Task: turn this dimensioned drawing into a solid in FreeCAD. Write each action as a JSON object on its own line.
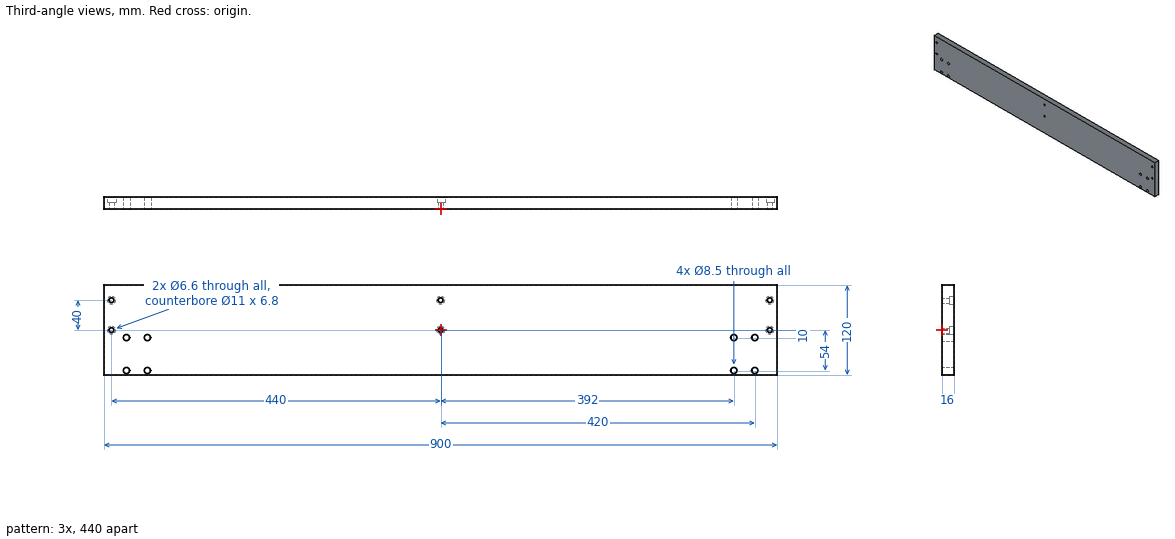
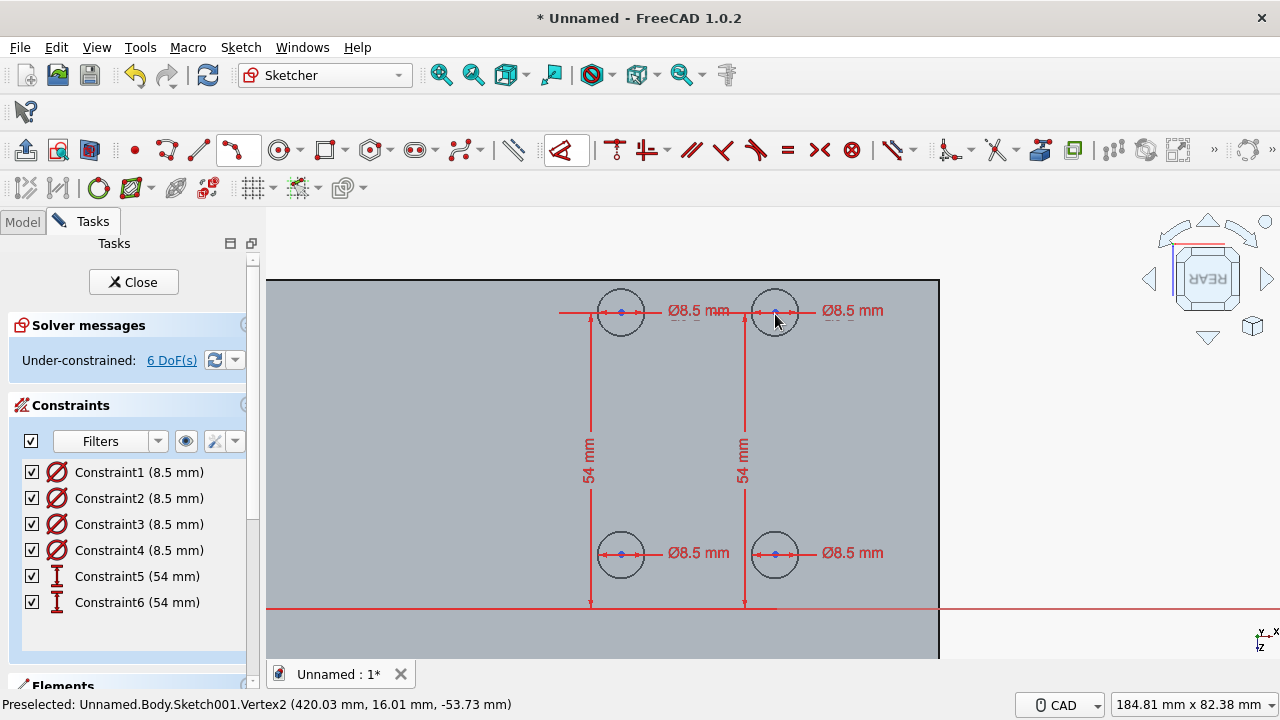
{"action": "left_click", "coordinate": [621, 555]}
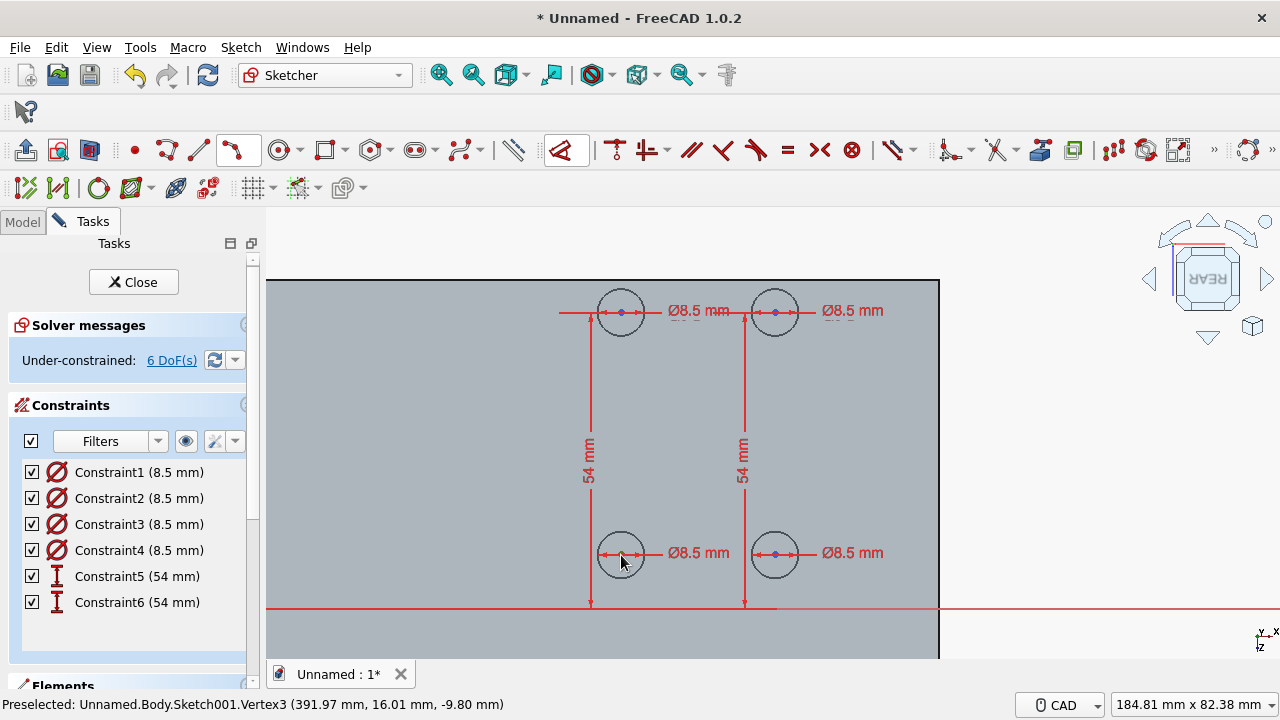
{"action": "left_click", "coordinate": [584, 150]}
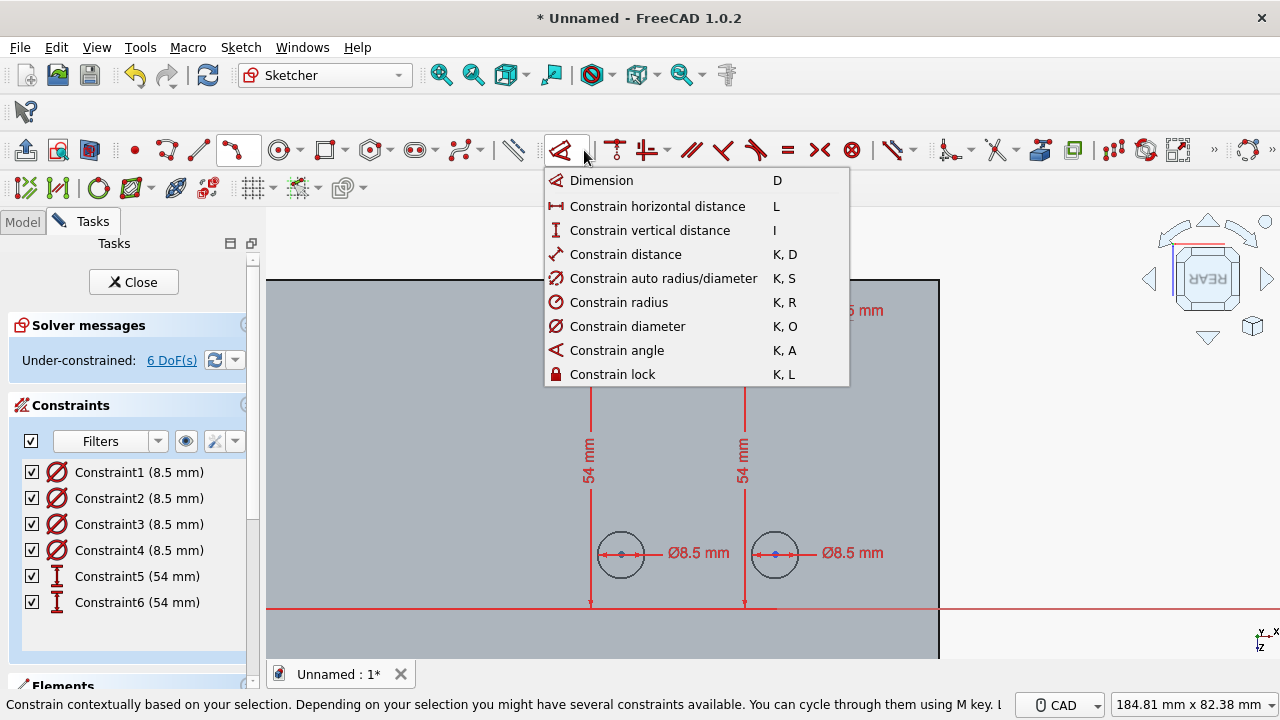
{"action": "left_click", "coordinate": [697, 230]}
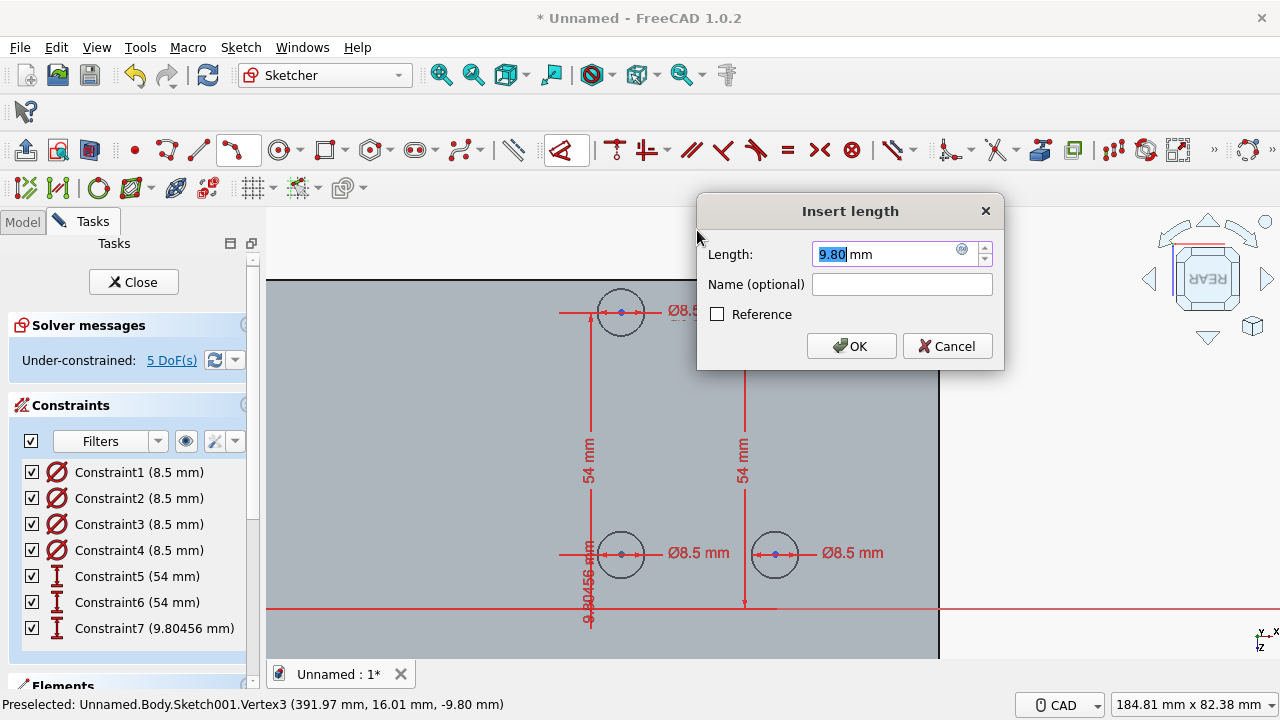
{"action": "type", "text": "10"}
{"action": "key", "text": "Return"}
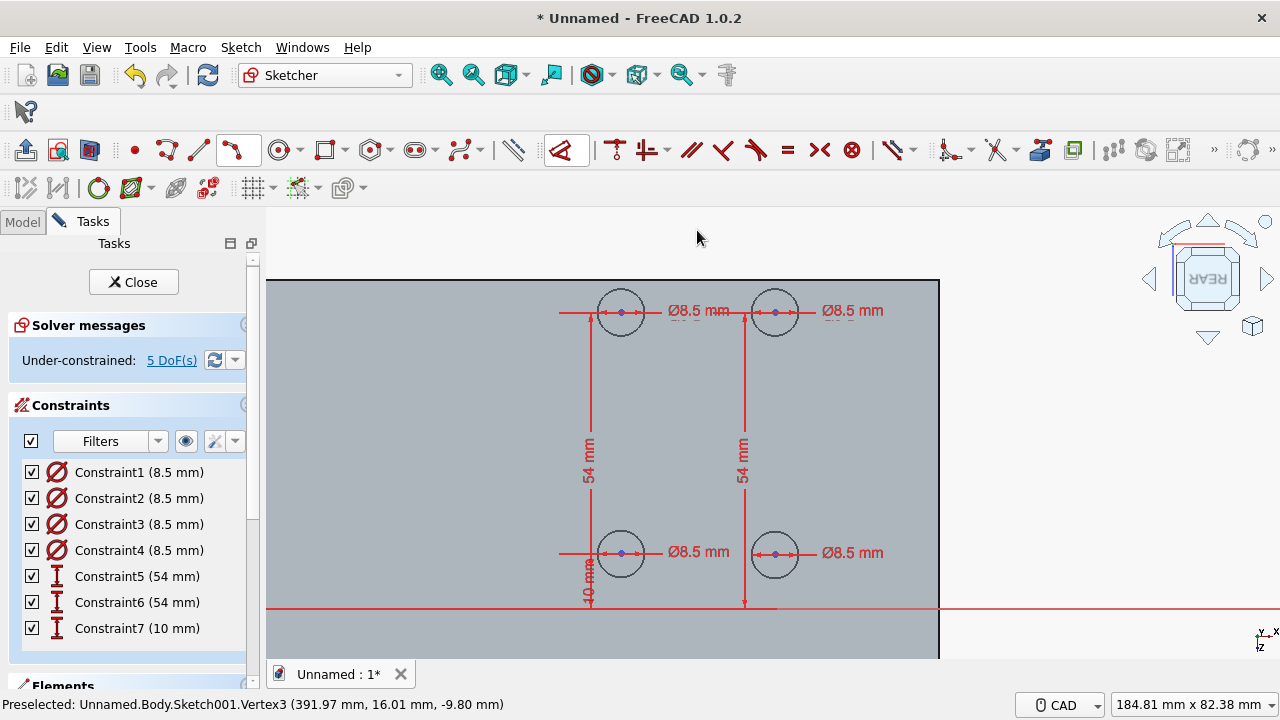
{"action": "left_click", "coordinate": [775, 555]}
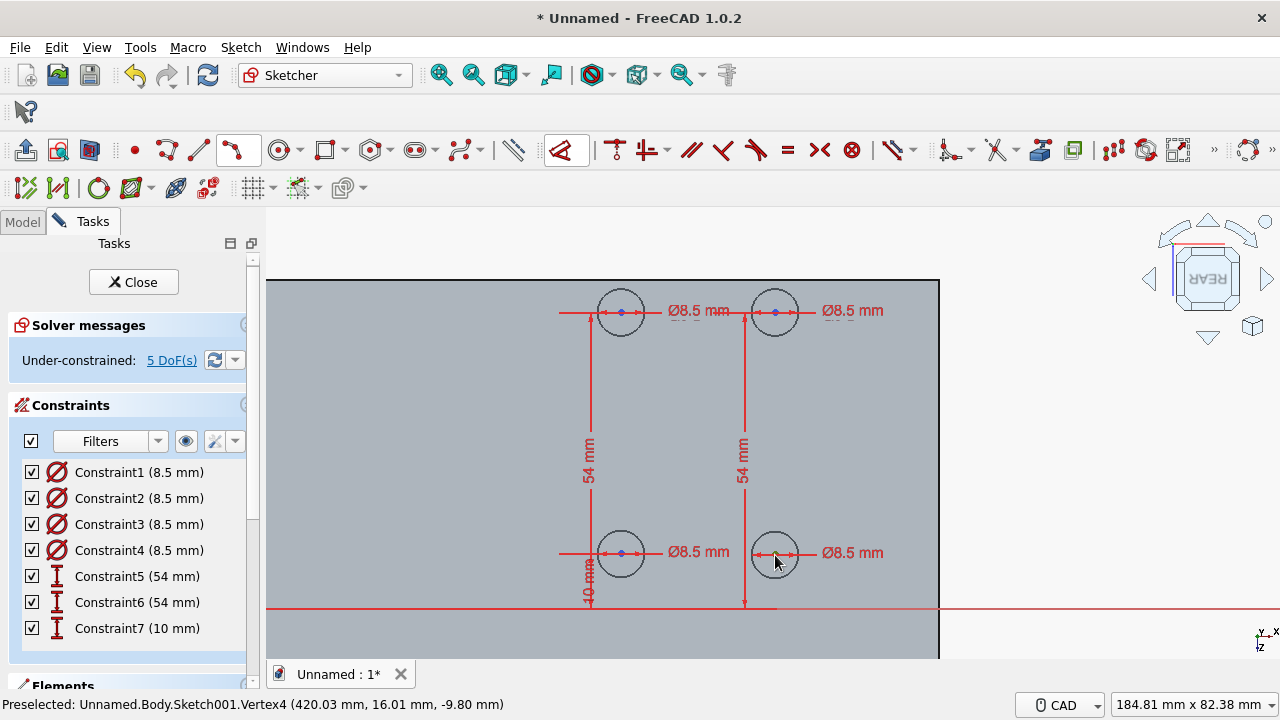
{"action": "key", "text": "i"}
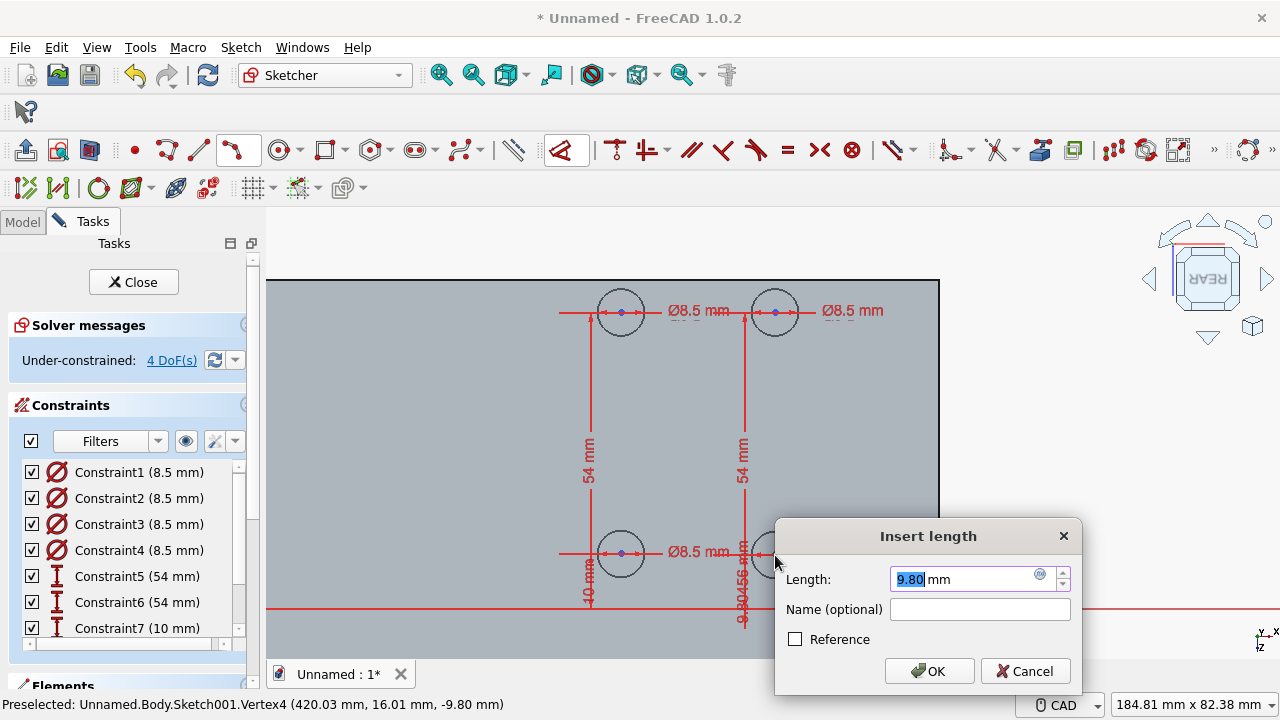
{"action": "type", "text": "10"}
{"action": "key", "text": "Return"}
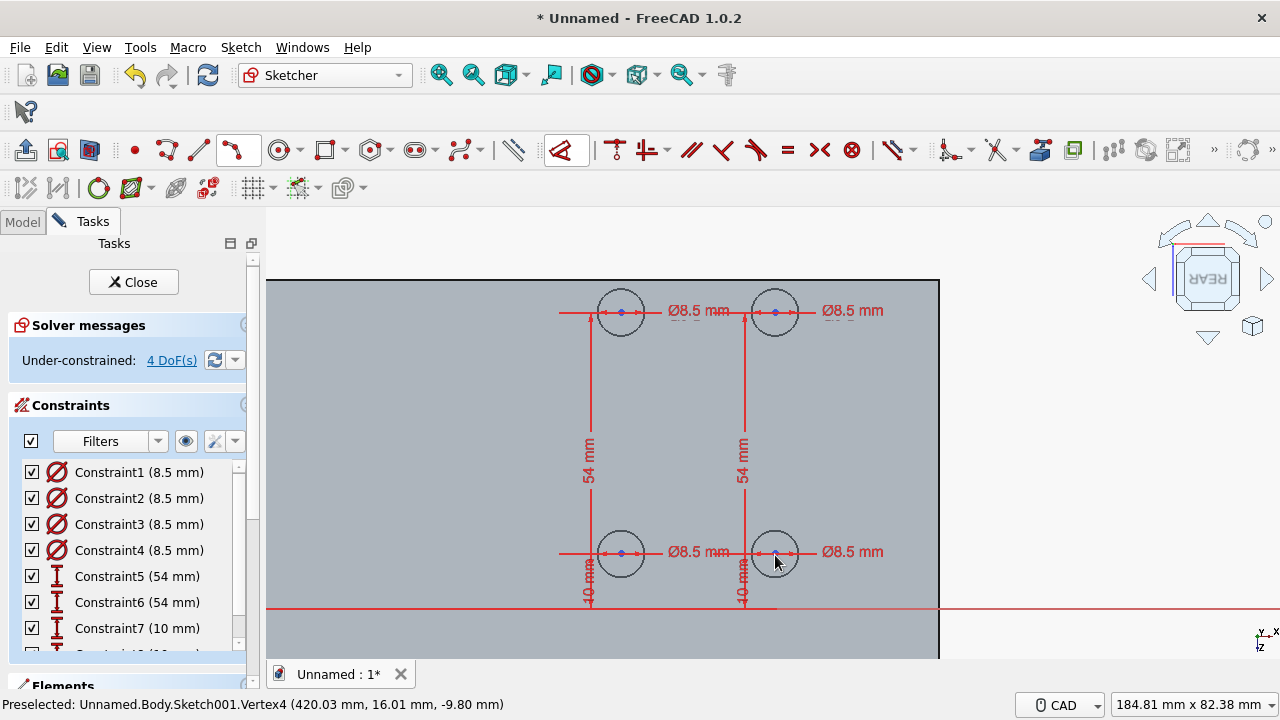
{"action": "left_click", "coordinate": [621, 313]}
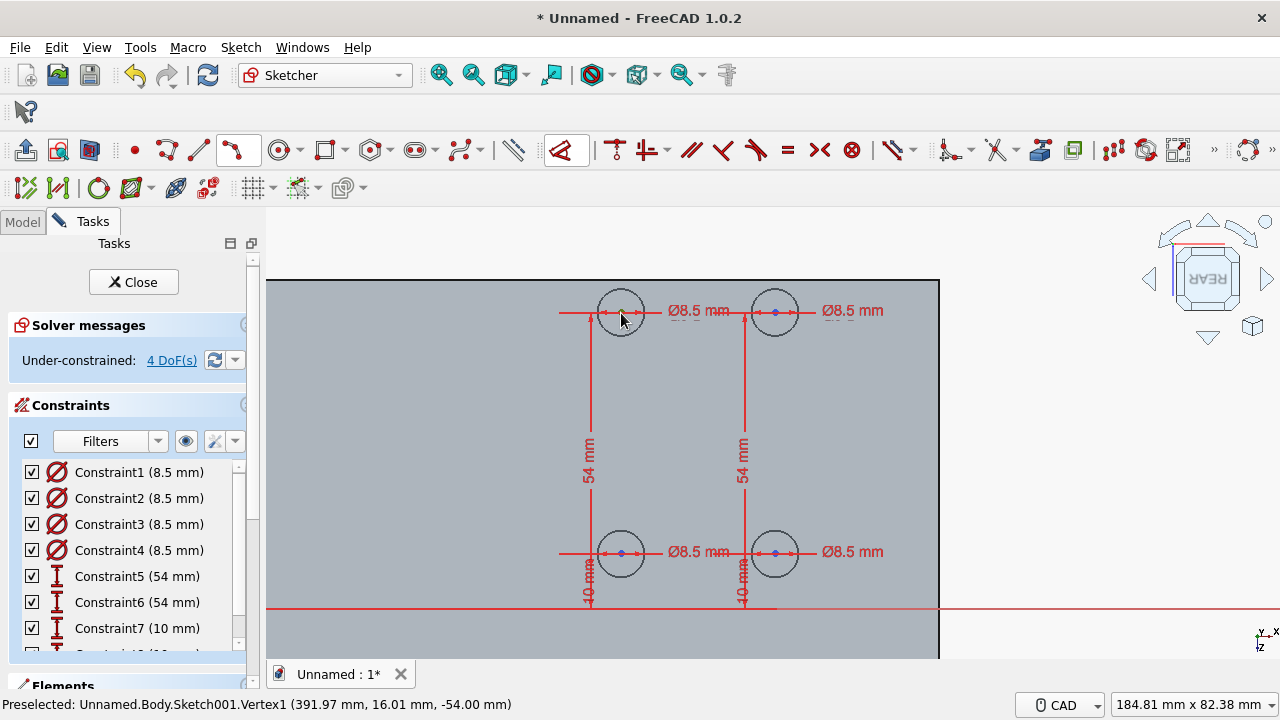
{"action": "key", "text": "l"}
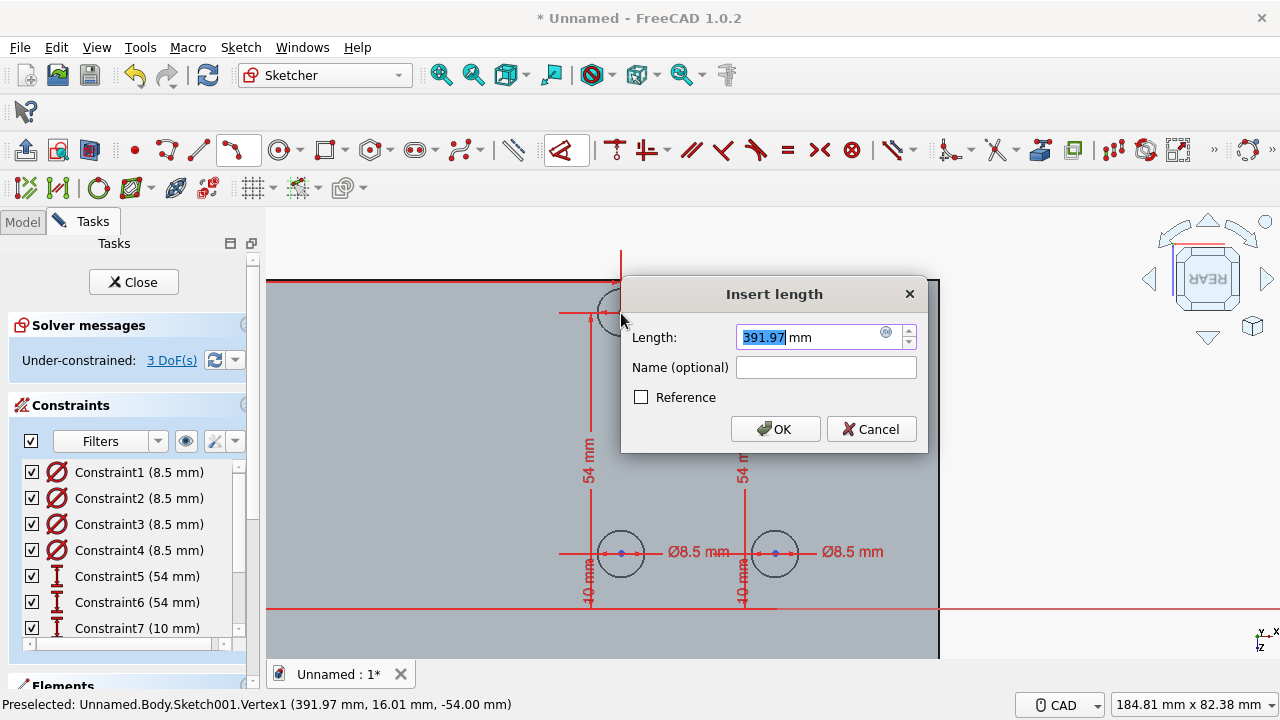
{"action": "type", "text": "392"}
{"action": "key", "text": "Return"}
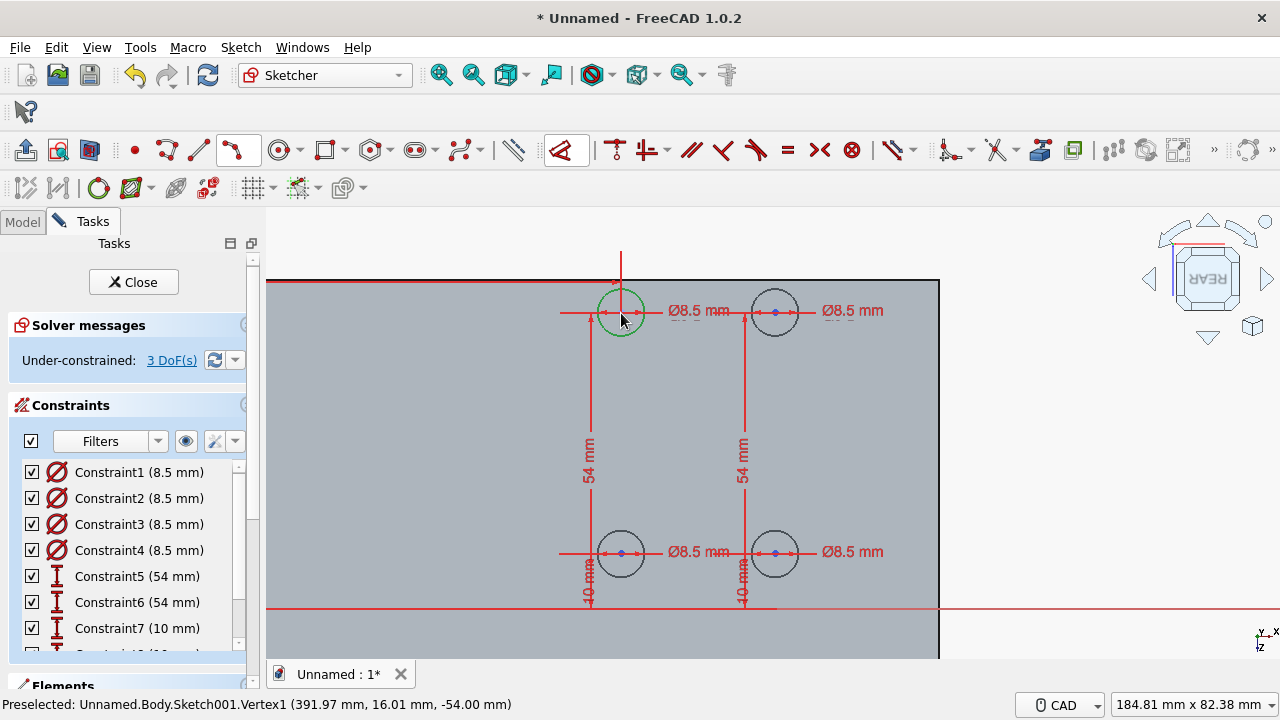
{"action": "left_click", "coordinate": [775, 313]}